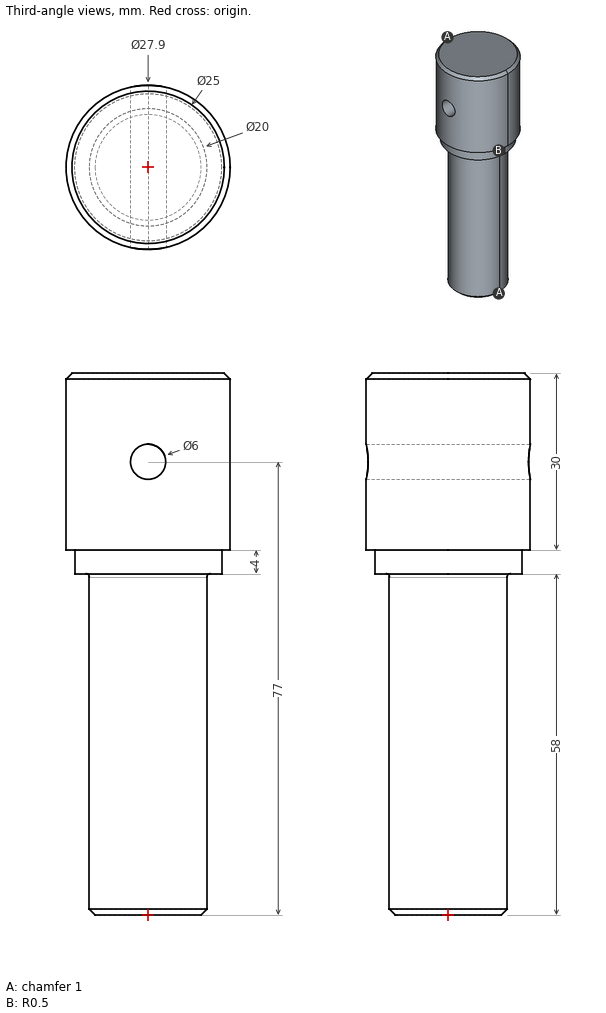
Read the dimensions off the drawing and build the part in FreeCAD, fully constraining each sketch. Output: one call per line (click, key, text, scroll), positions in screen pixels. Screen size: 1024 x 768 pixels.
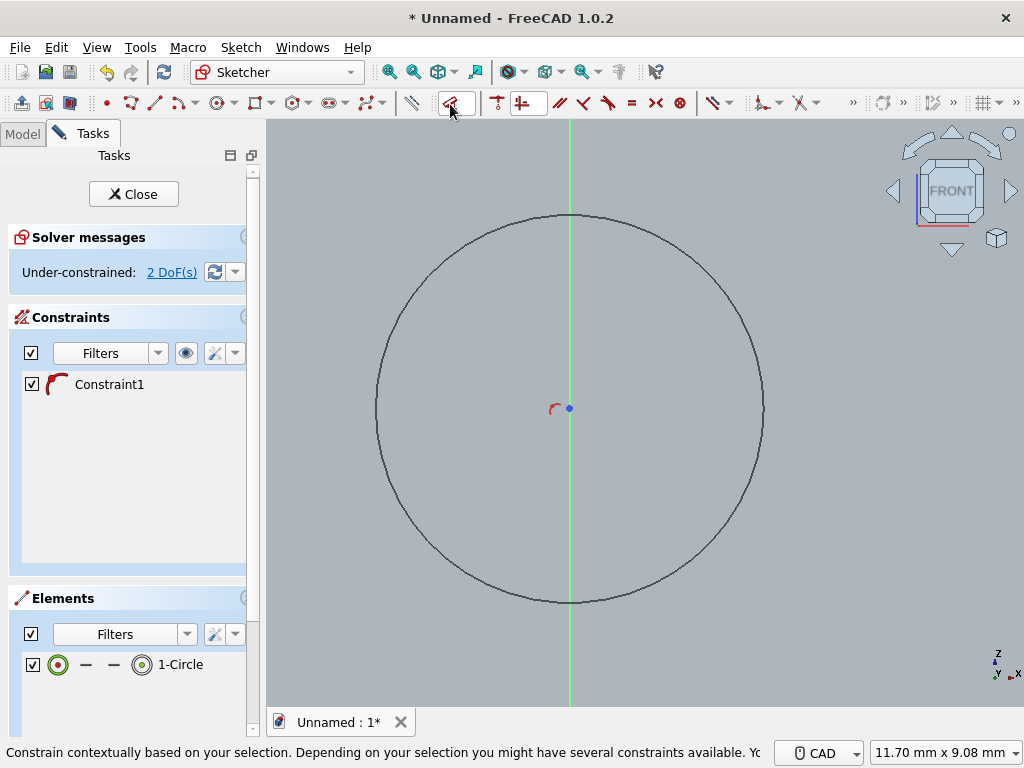
click(706, 271)
click(728, 248)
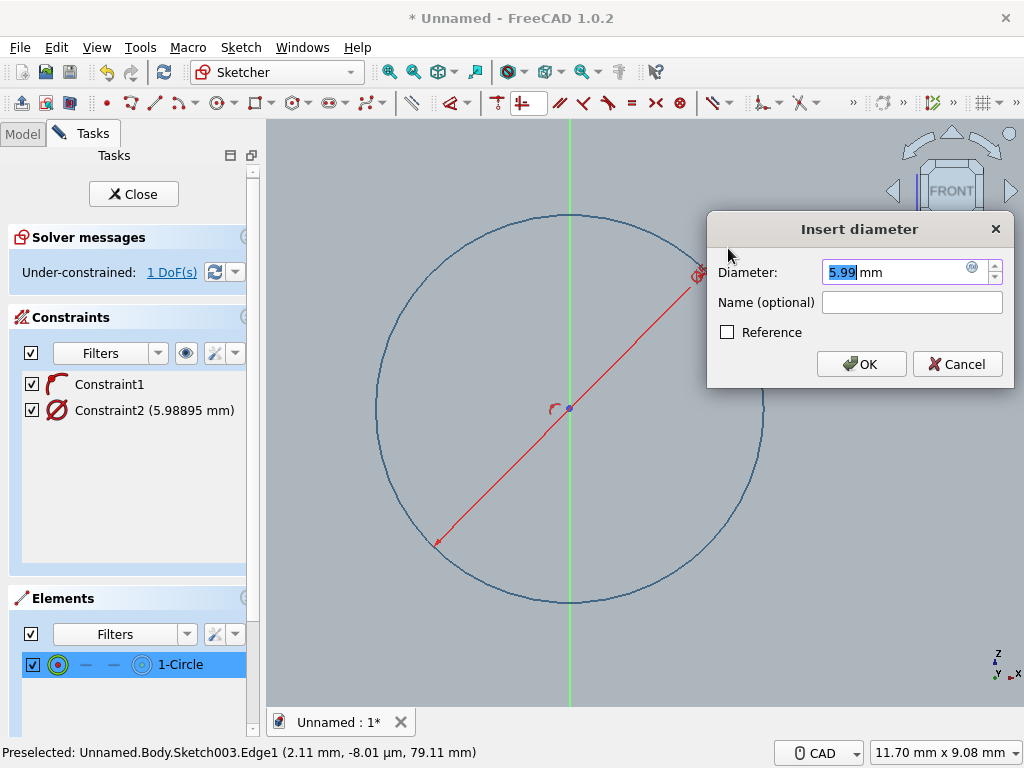
text(6)
key(Return)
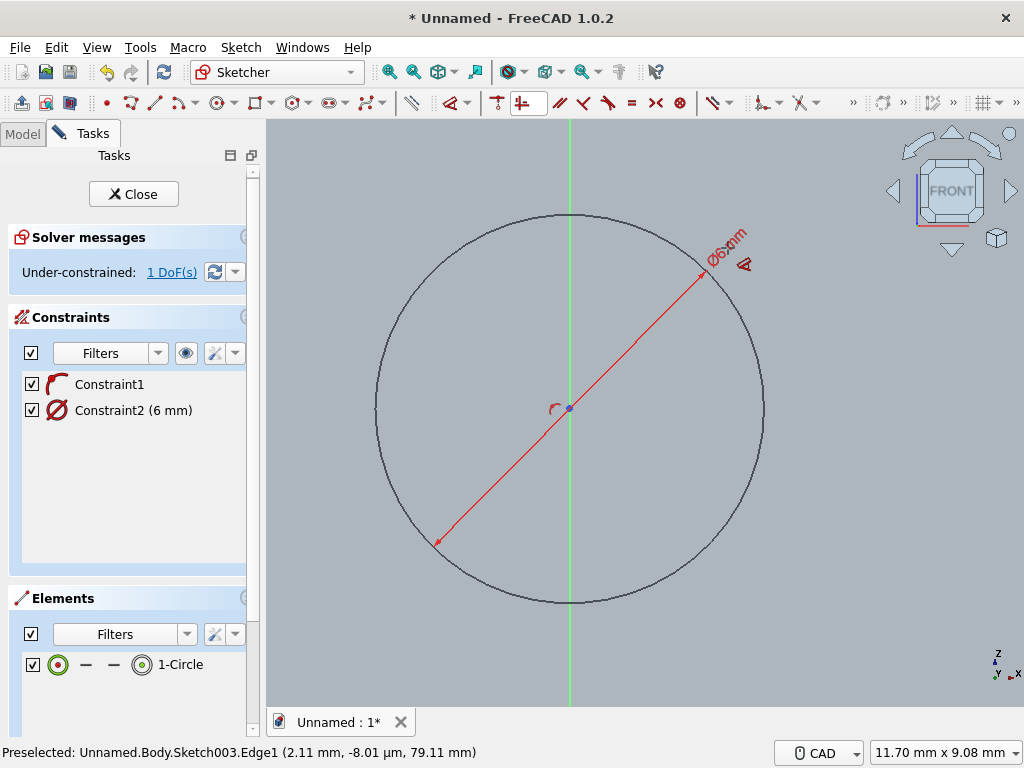
click(570, 409)
click(604, 544)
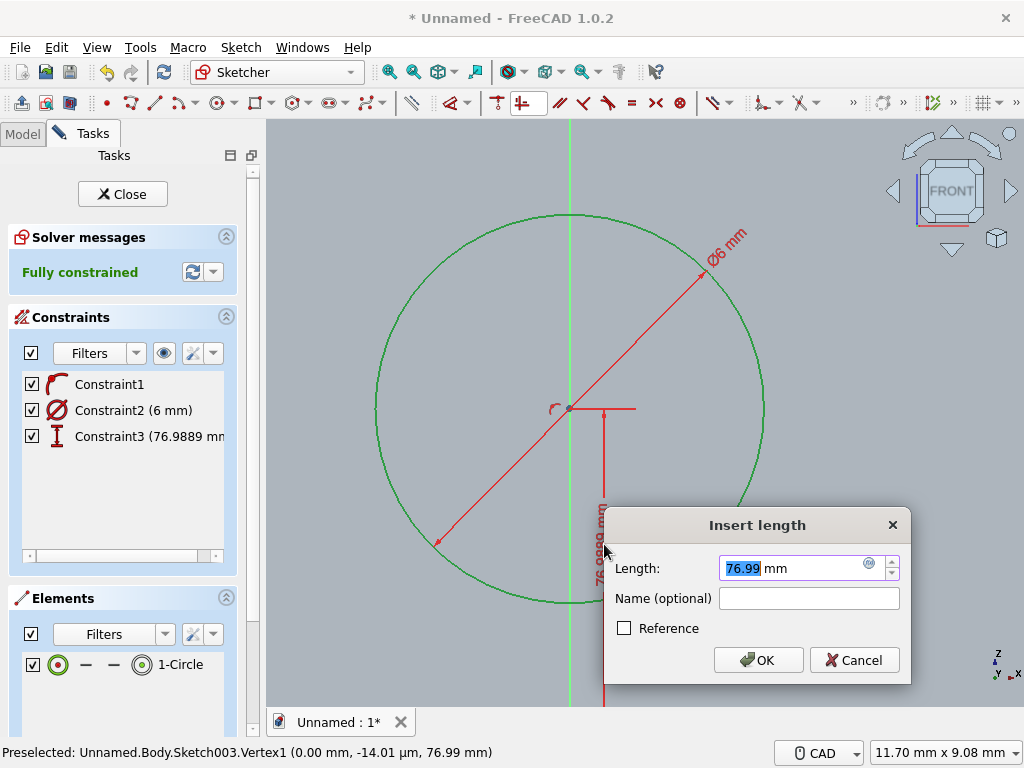
text(77)
key(Return)
key(Escape)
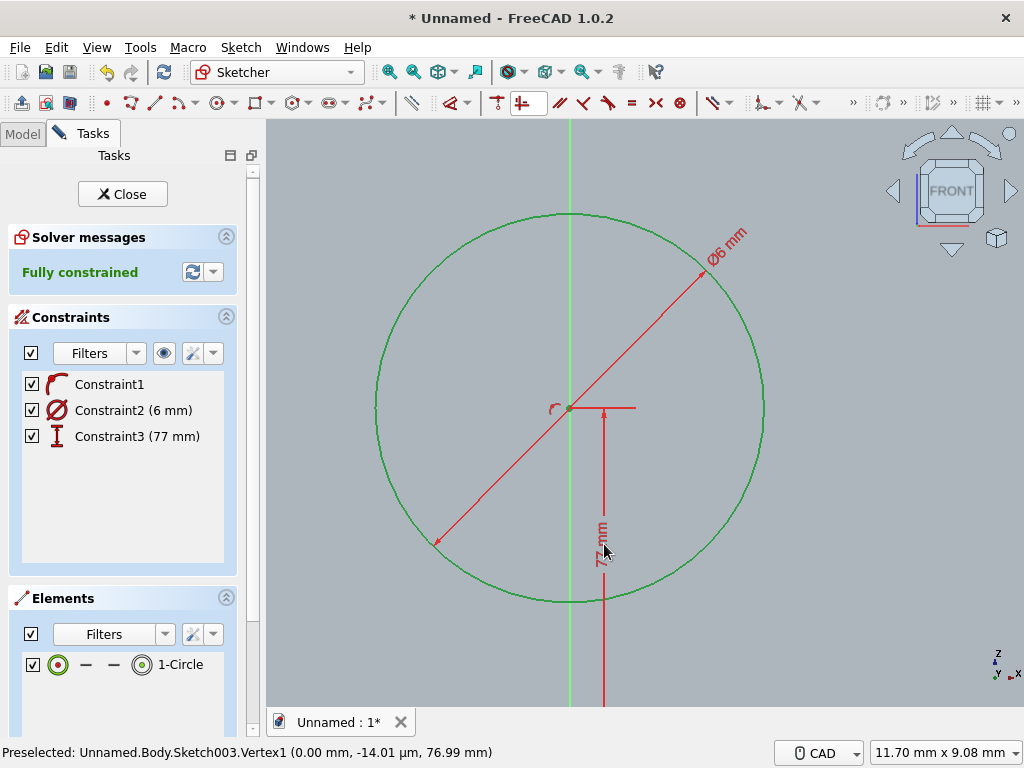
click(123, 194)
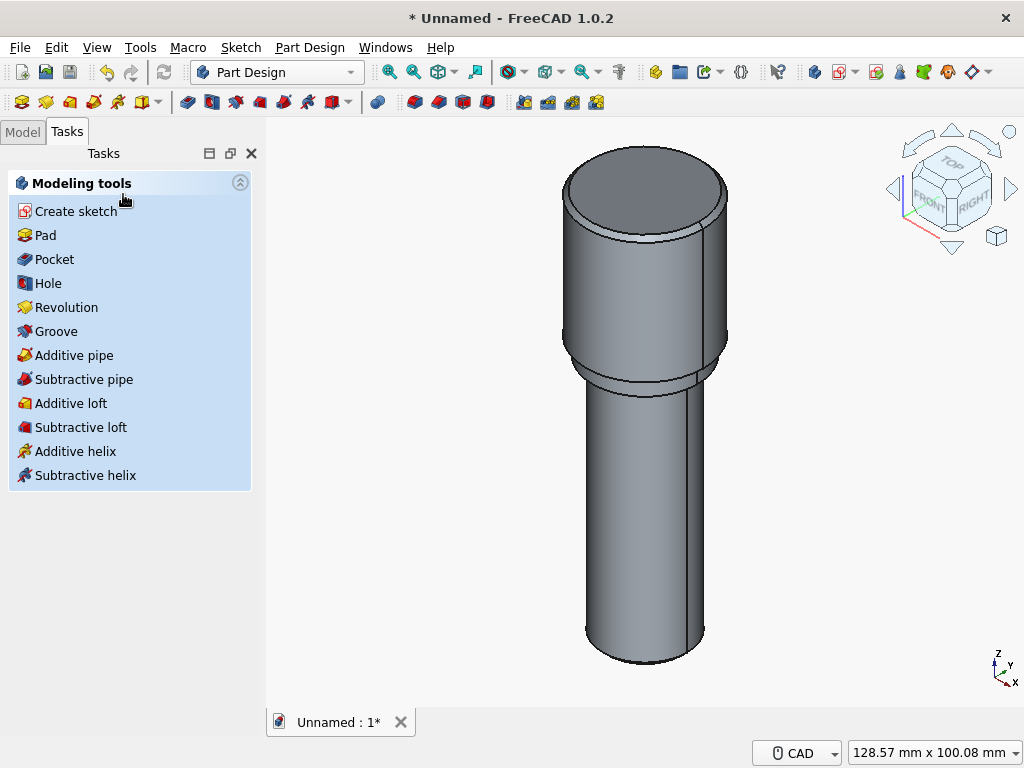
click(188, 102)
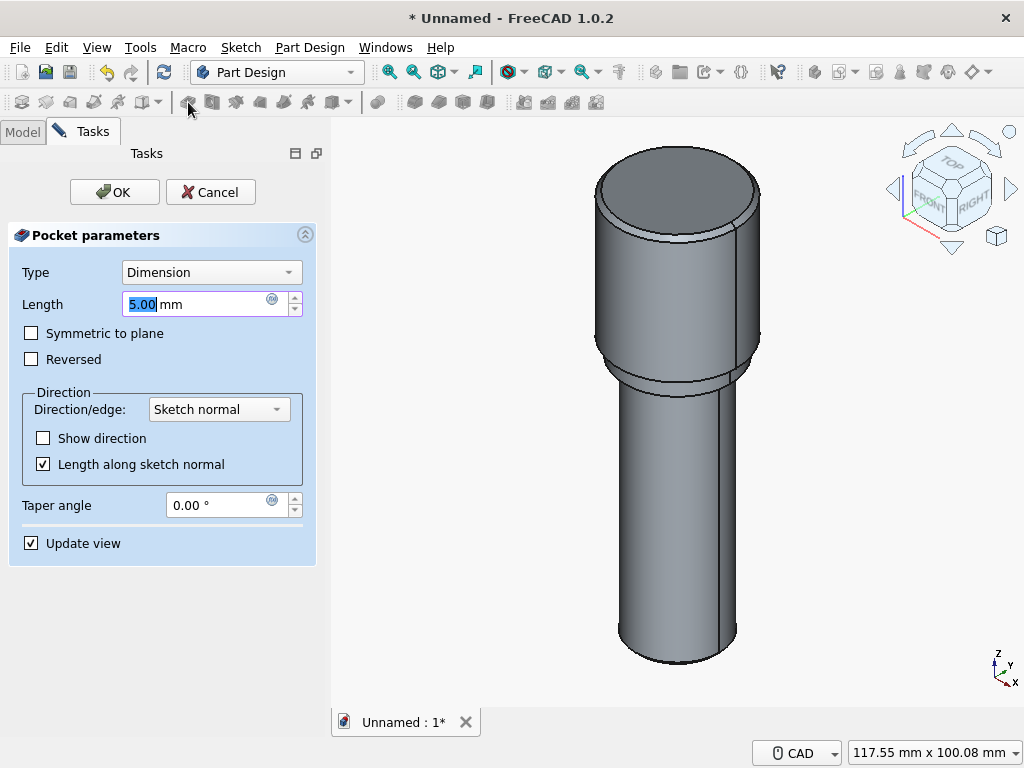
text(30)
key(Tab)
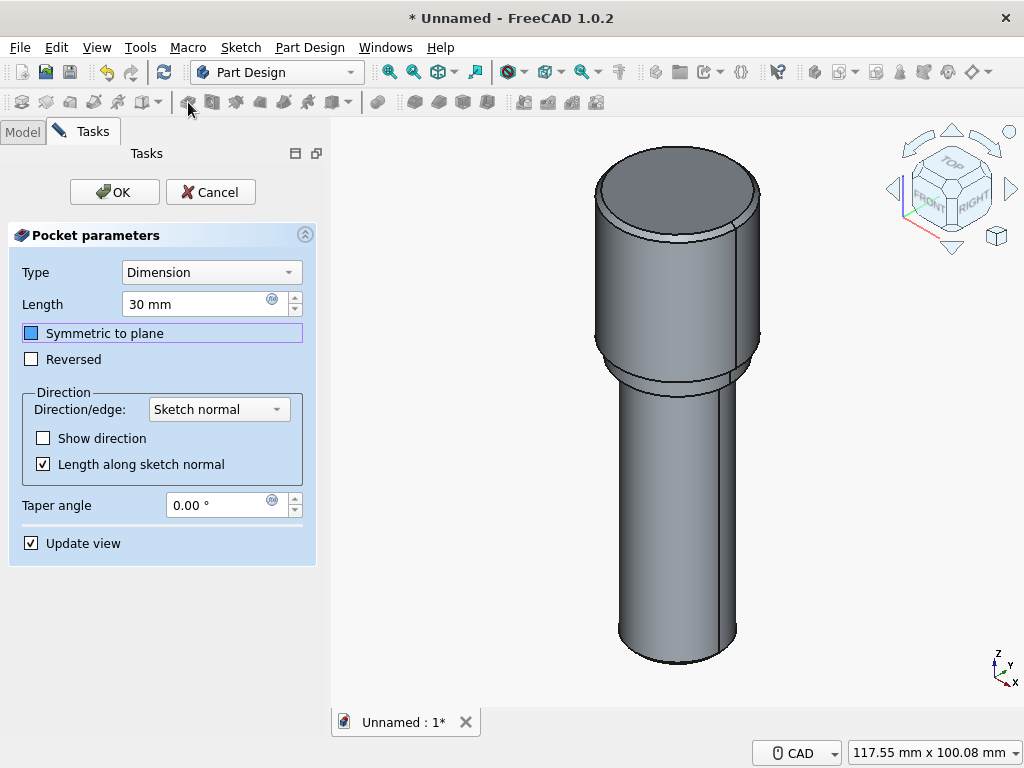
click(30, 333)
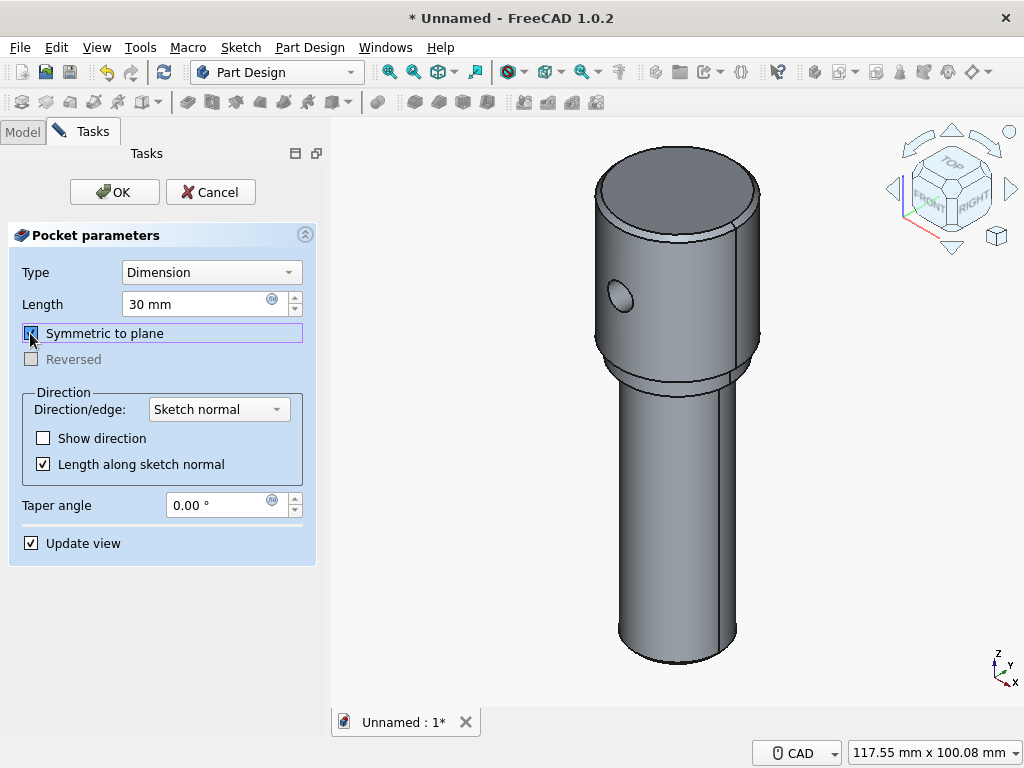
click(115, 192)